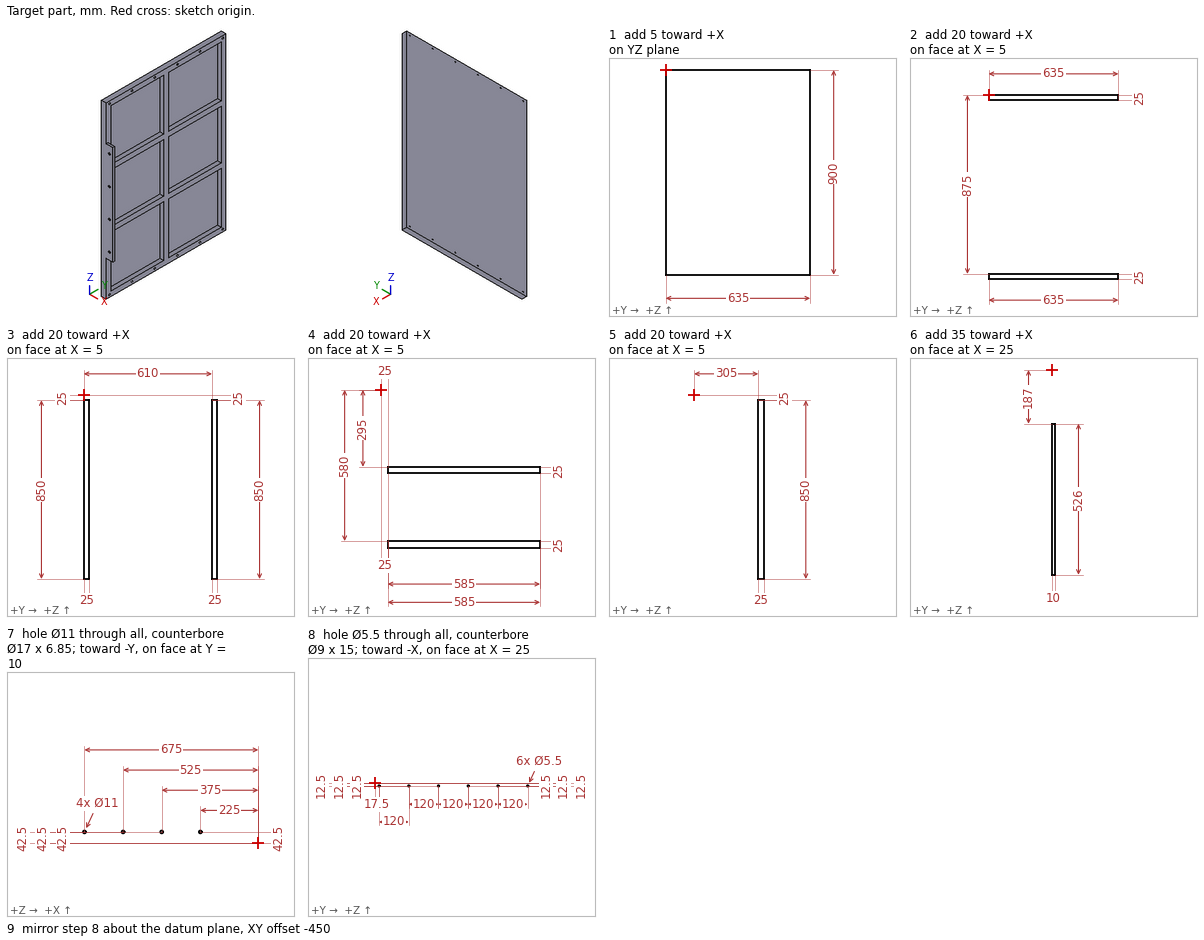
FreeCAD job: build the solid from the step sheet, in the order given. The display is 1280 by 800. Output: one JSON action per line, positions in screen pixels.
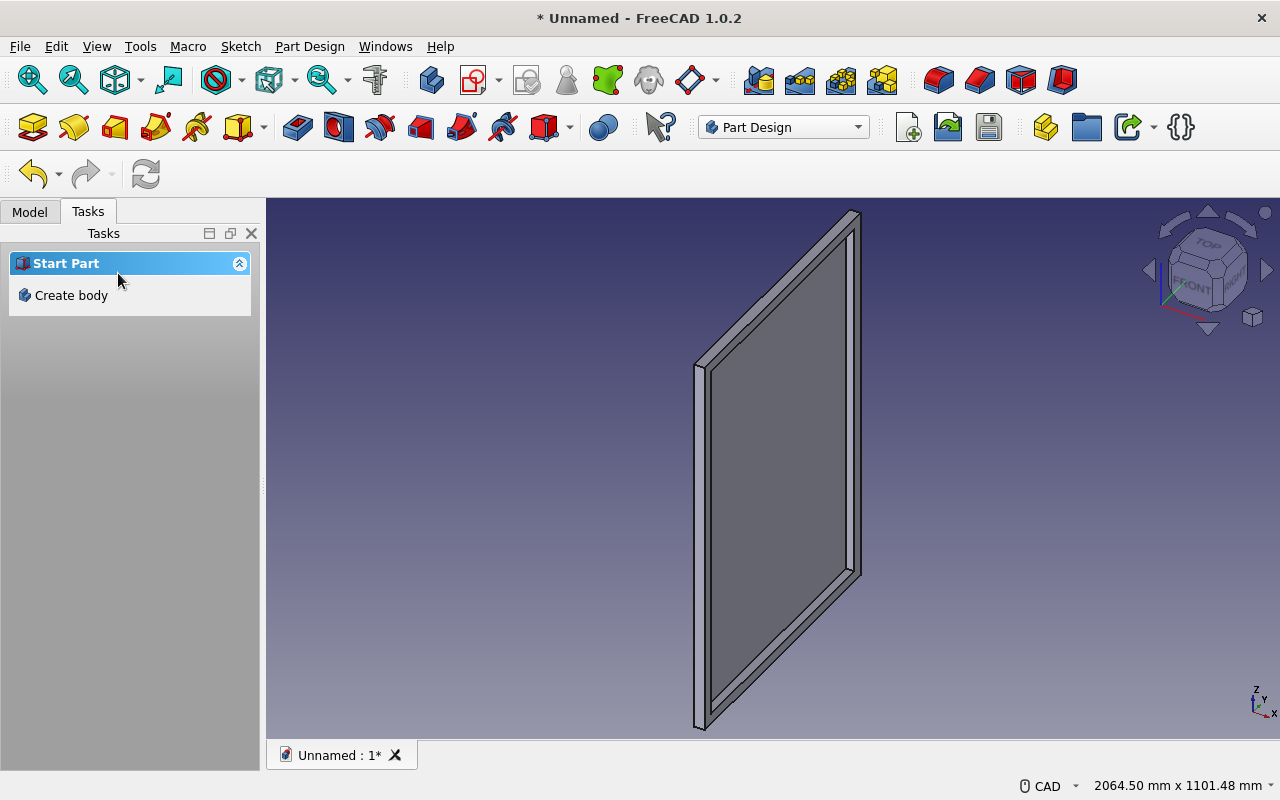
{"action": "left_click", "coordinate": [774, 468]}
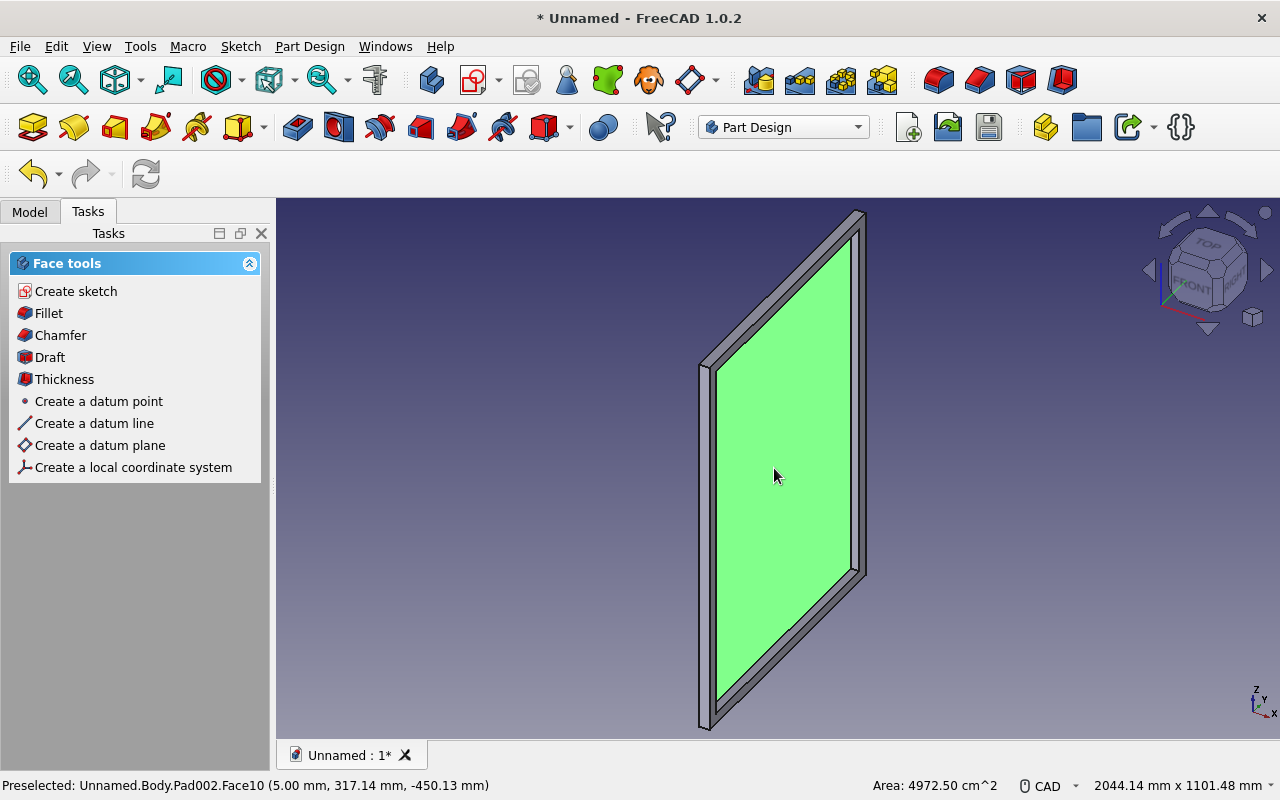
{"action": "left_click", "coordinate": [472, 80]}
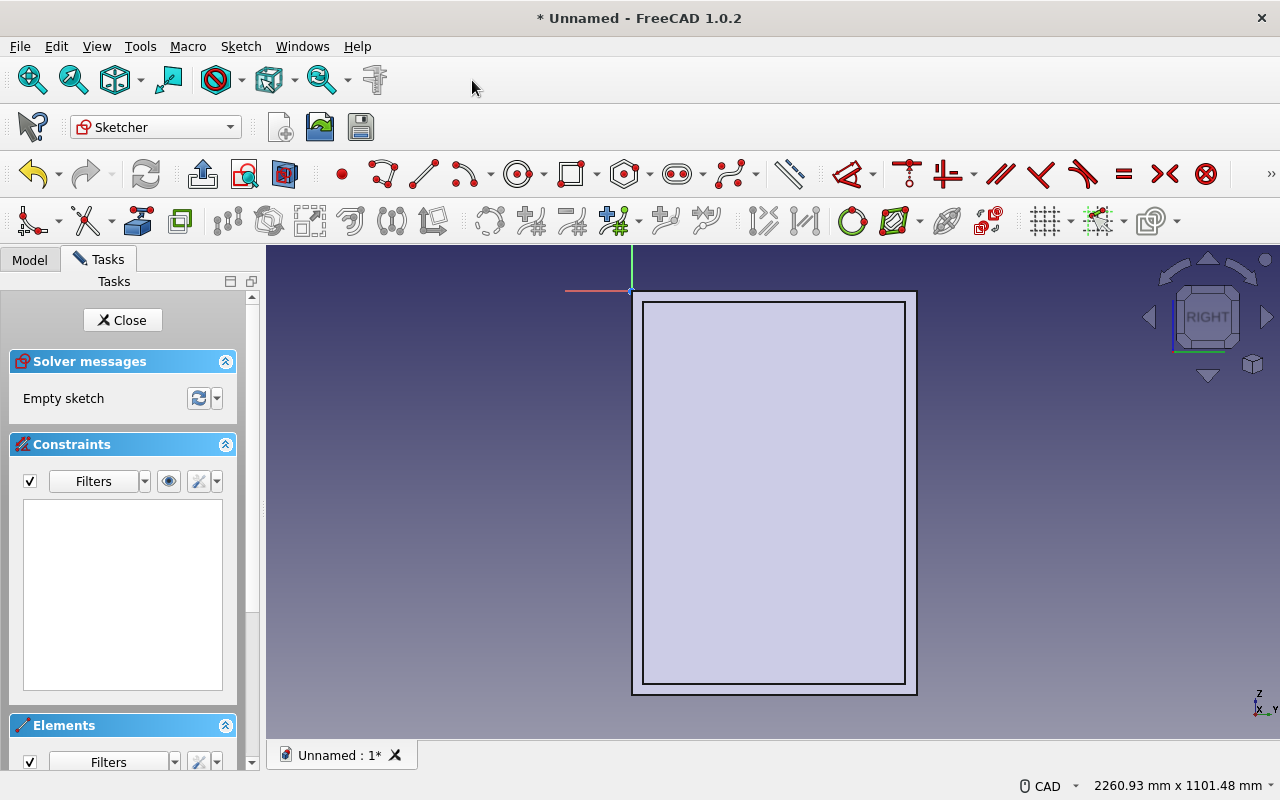
{"action": "left_click", "coordinate": [285, 174]}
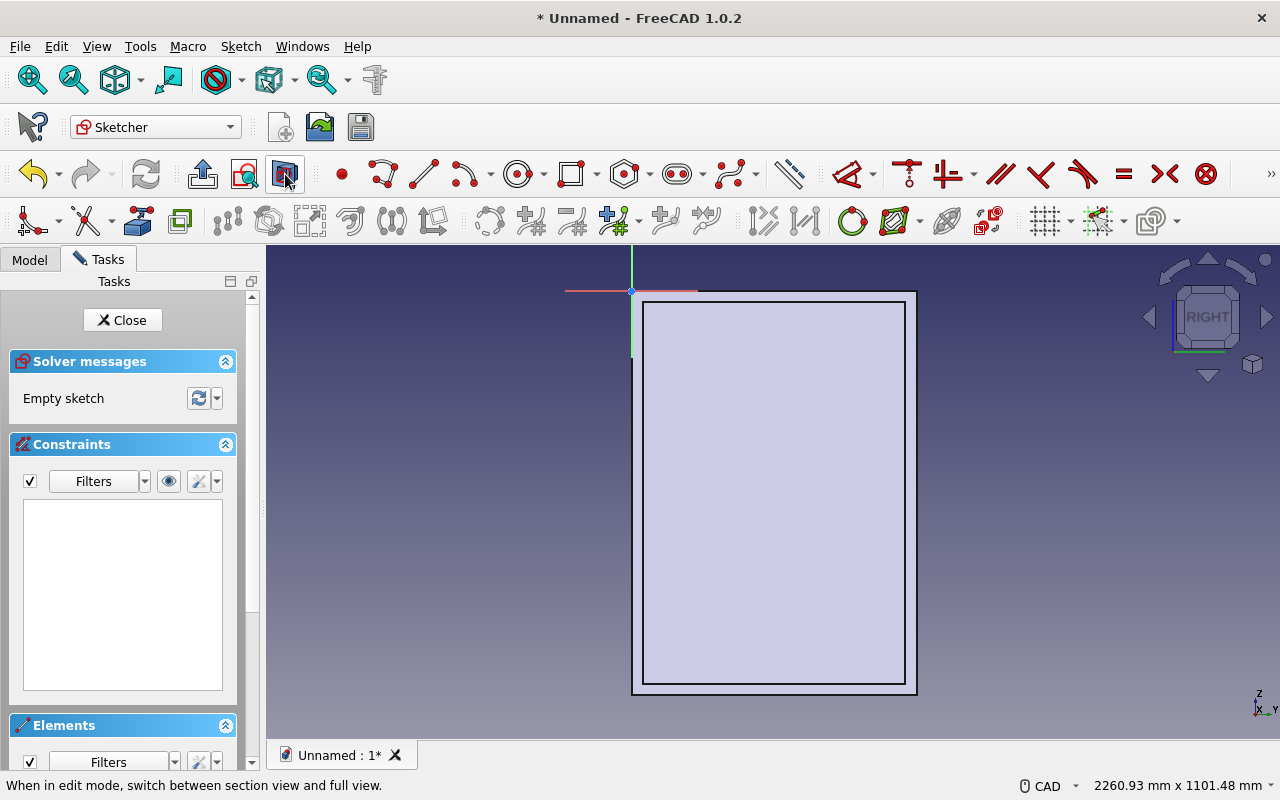
{"action": "scroll", "coordinate": [415, 711], "scroll_direction": "down", "scroll_amount": 1}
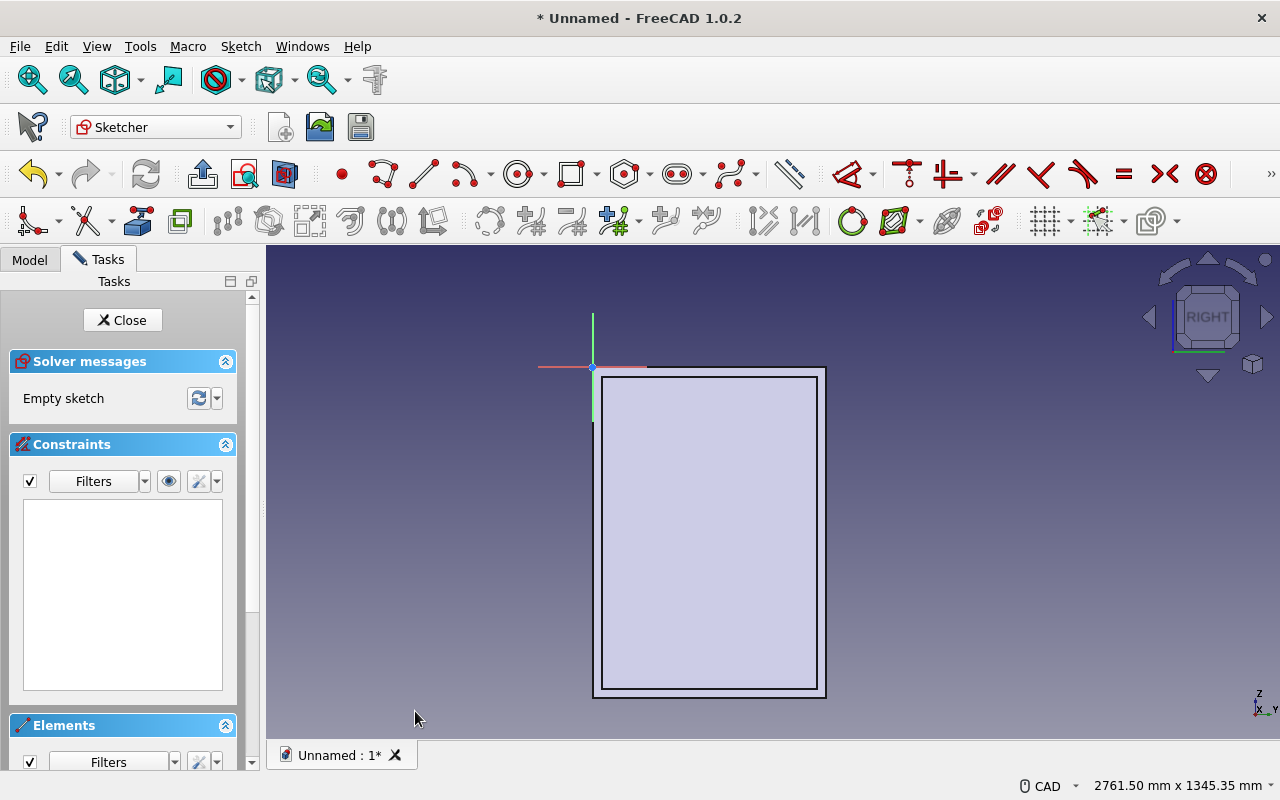
{"action": "scroll", "coordinate": [705, 451], "scroll_direction": "up", "scroll_amount": 2}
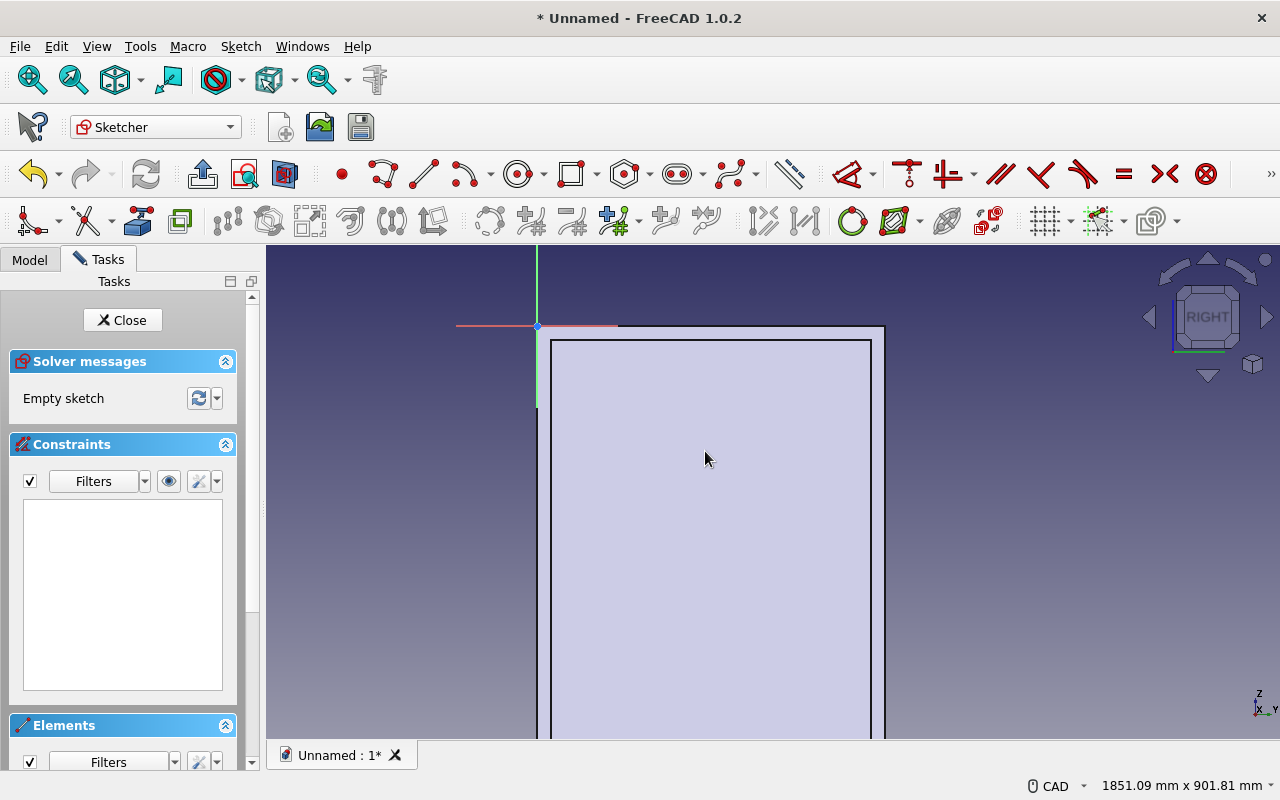
{"action": "key", "text": "g r"}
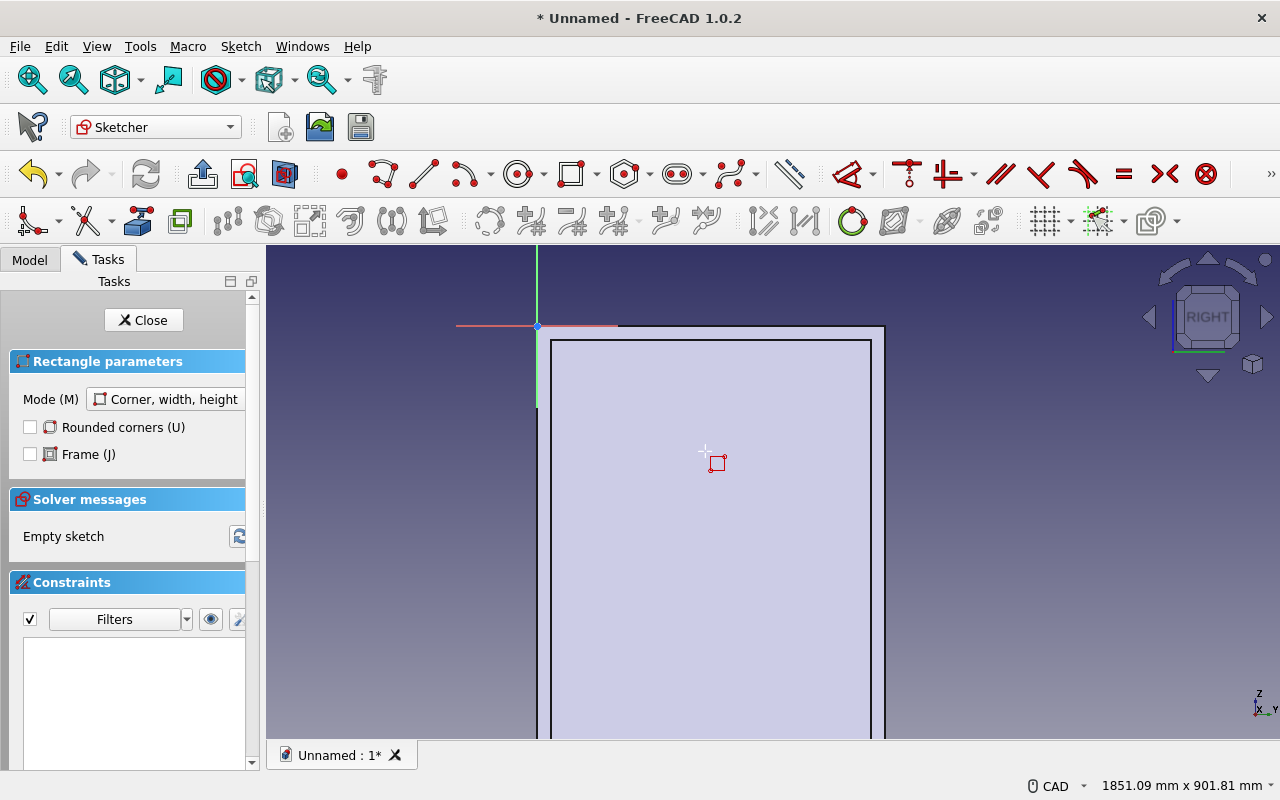
{"action": "left_click", "coordinate": [551, 488]}
{"action": "mouse_move", "coordinate": [871, 501]}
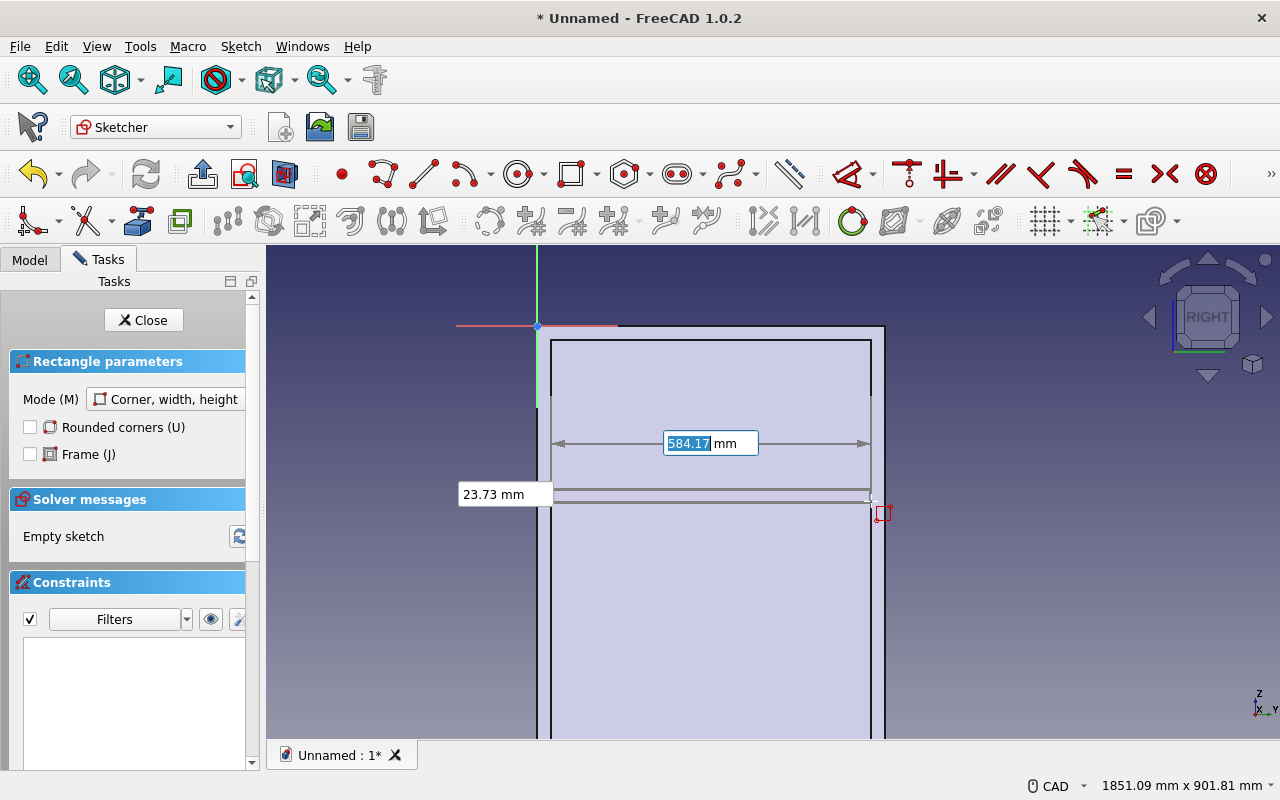
{"action": "type", "text": "585"}
{"action": "key", "text": "Tab"}
{"action": "type", "text": "25"}
{"action": "key", "text": "Return"}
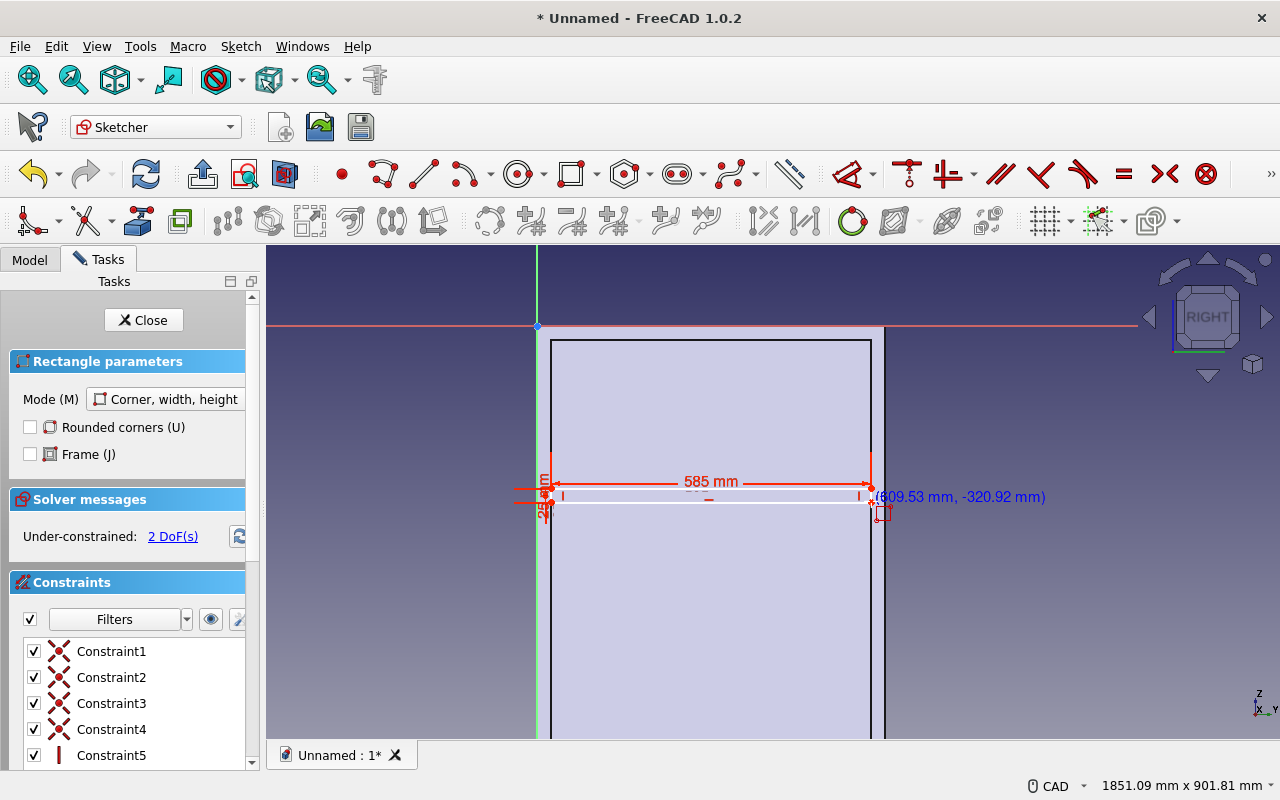
{"action": "left_click", "coordinate": [551, 644]}
{"action": "mouse_move", "coordinate": [871, 658]}